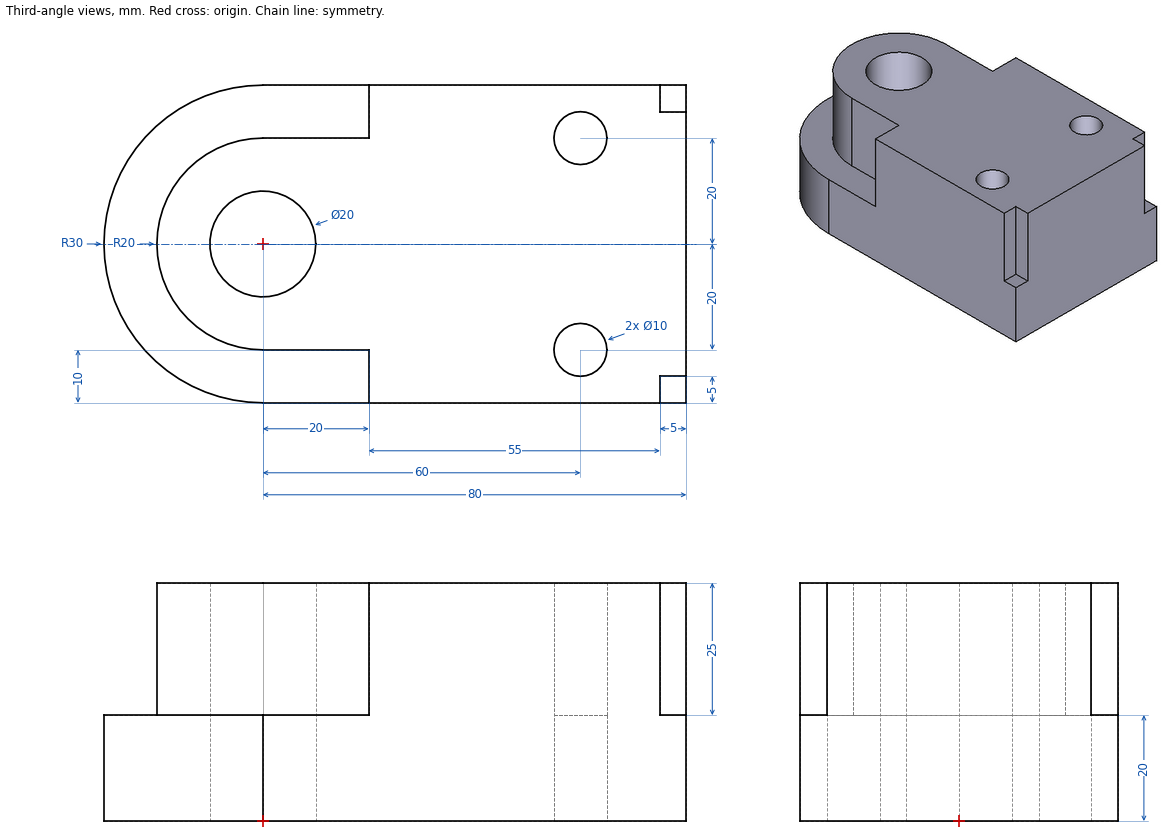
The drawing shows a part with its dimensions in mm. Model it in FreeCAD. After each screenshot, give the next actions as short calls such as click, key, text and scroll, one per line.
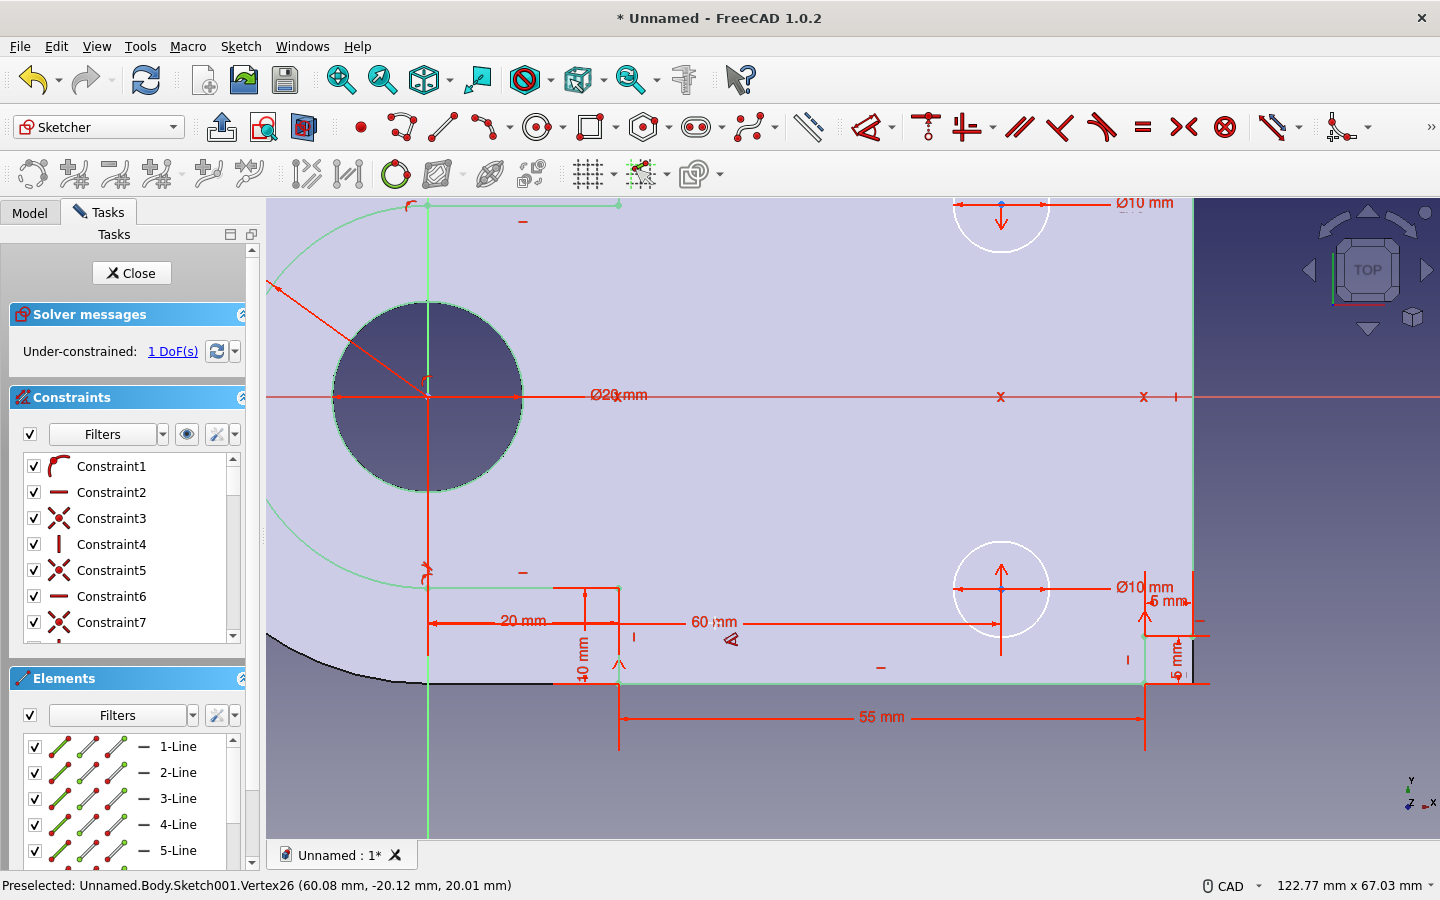
click(1001, 589)
click(1035, 493)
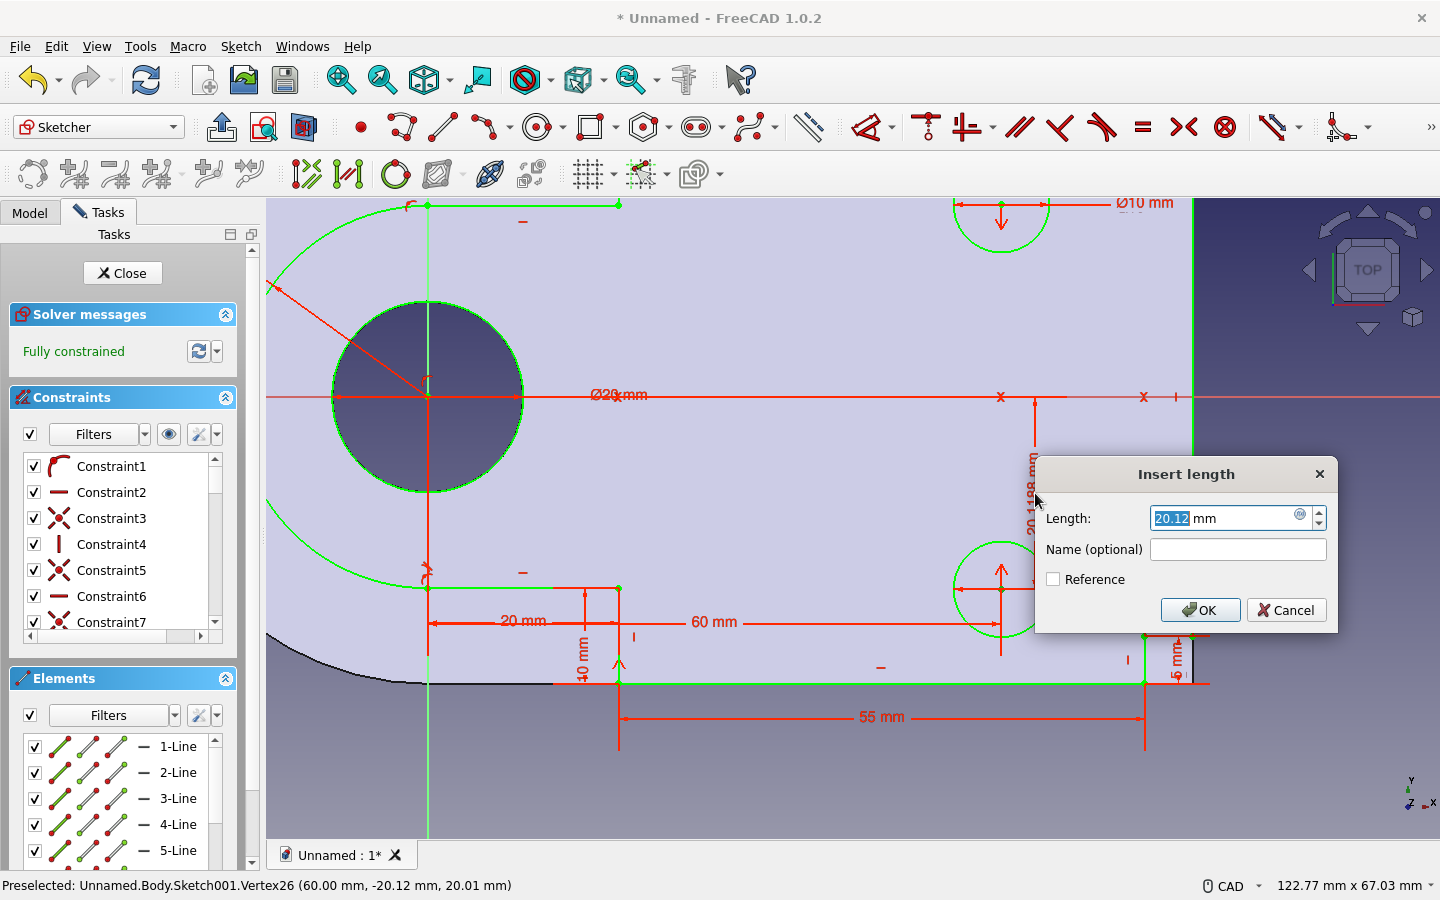
text(20)
key(Return)
key(Escape)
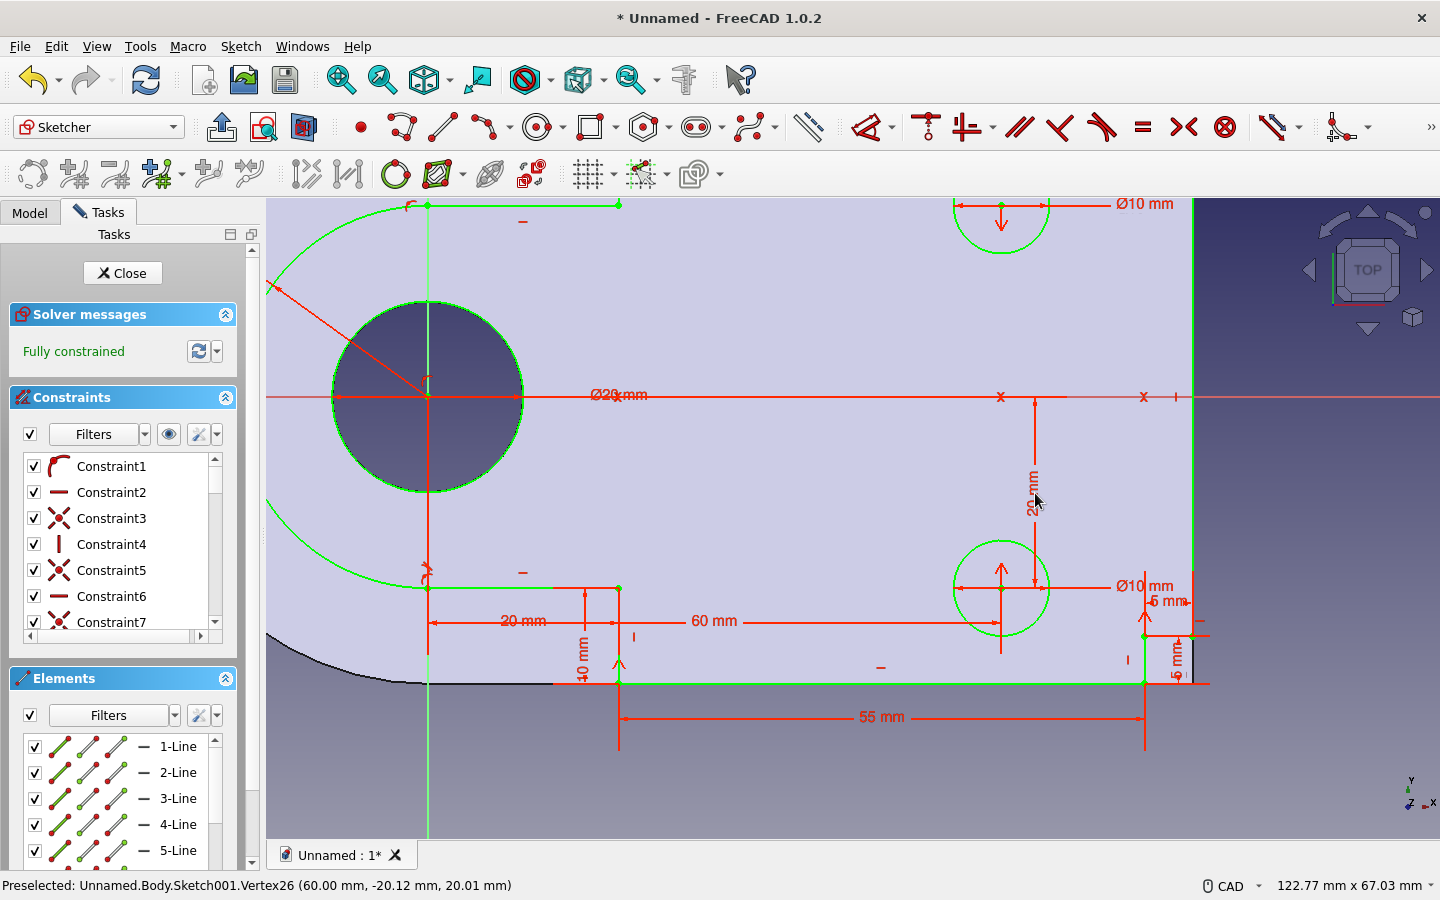
click(123, 273)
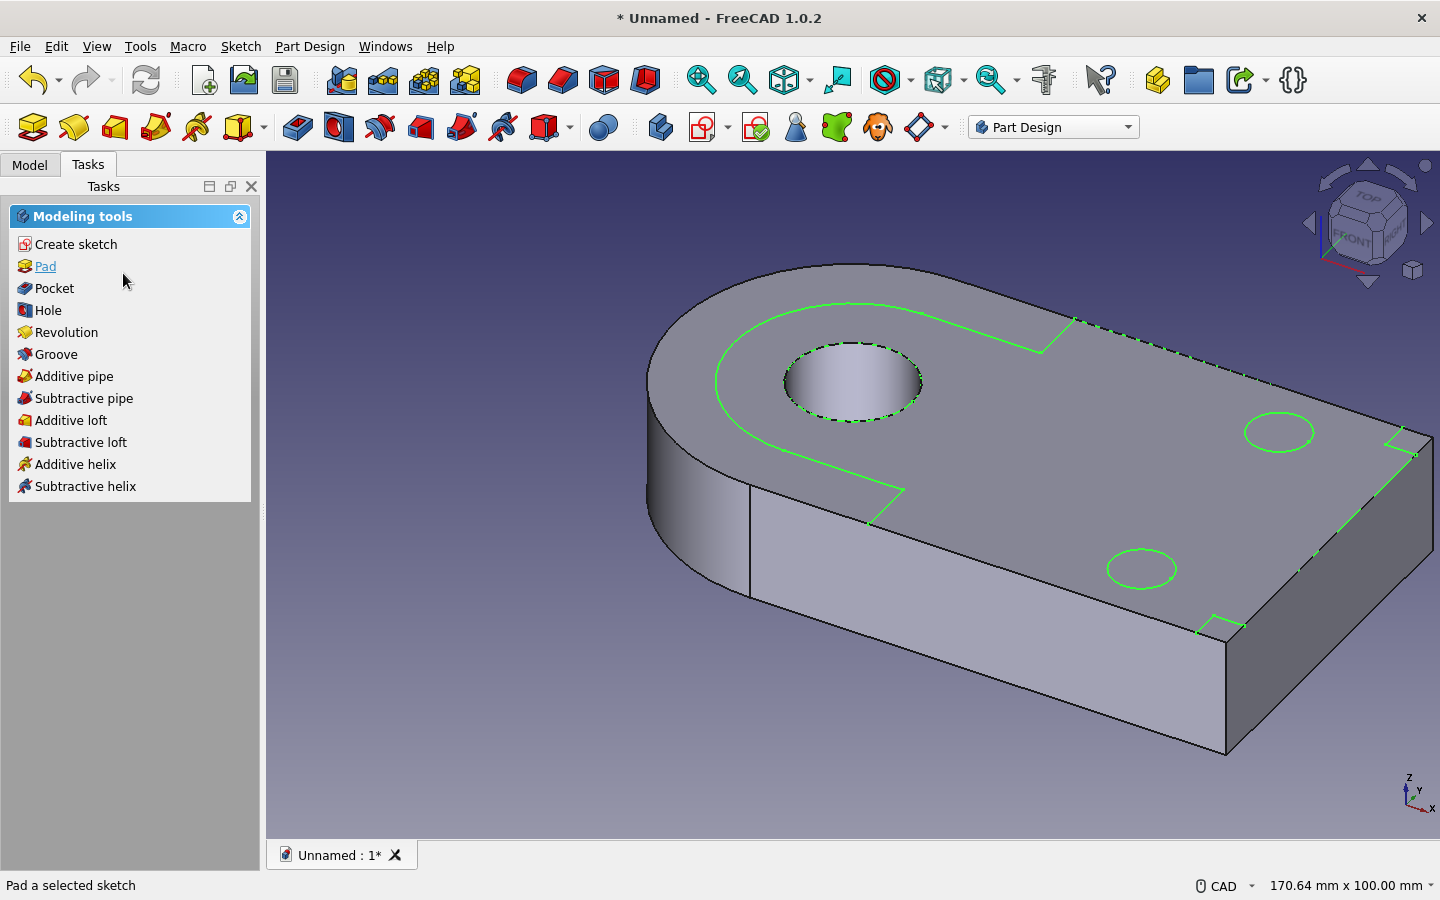
click(33, 128)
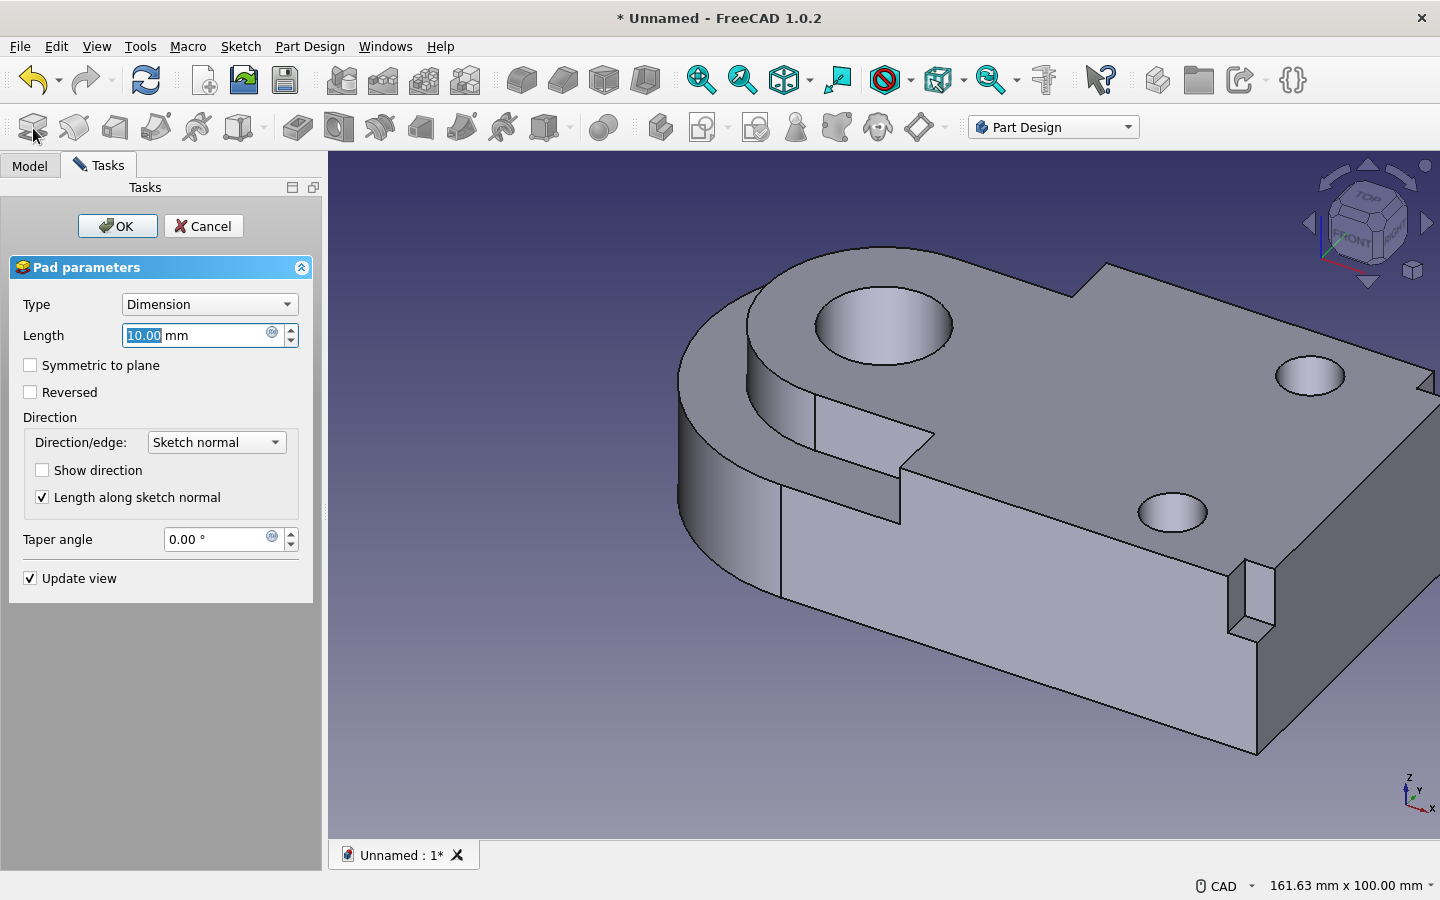
text(25)
key(Tab)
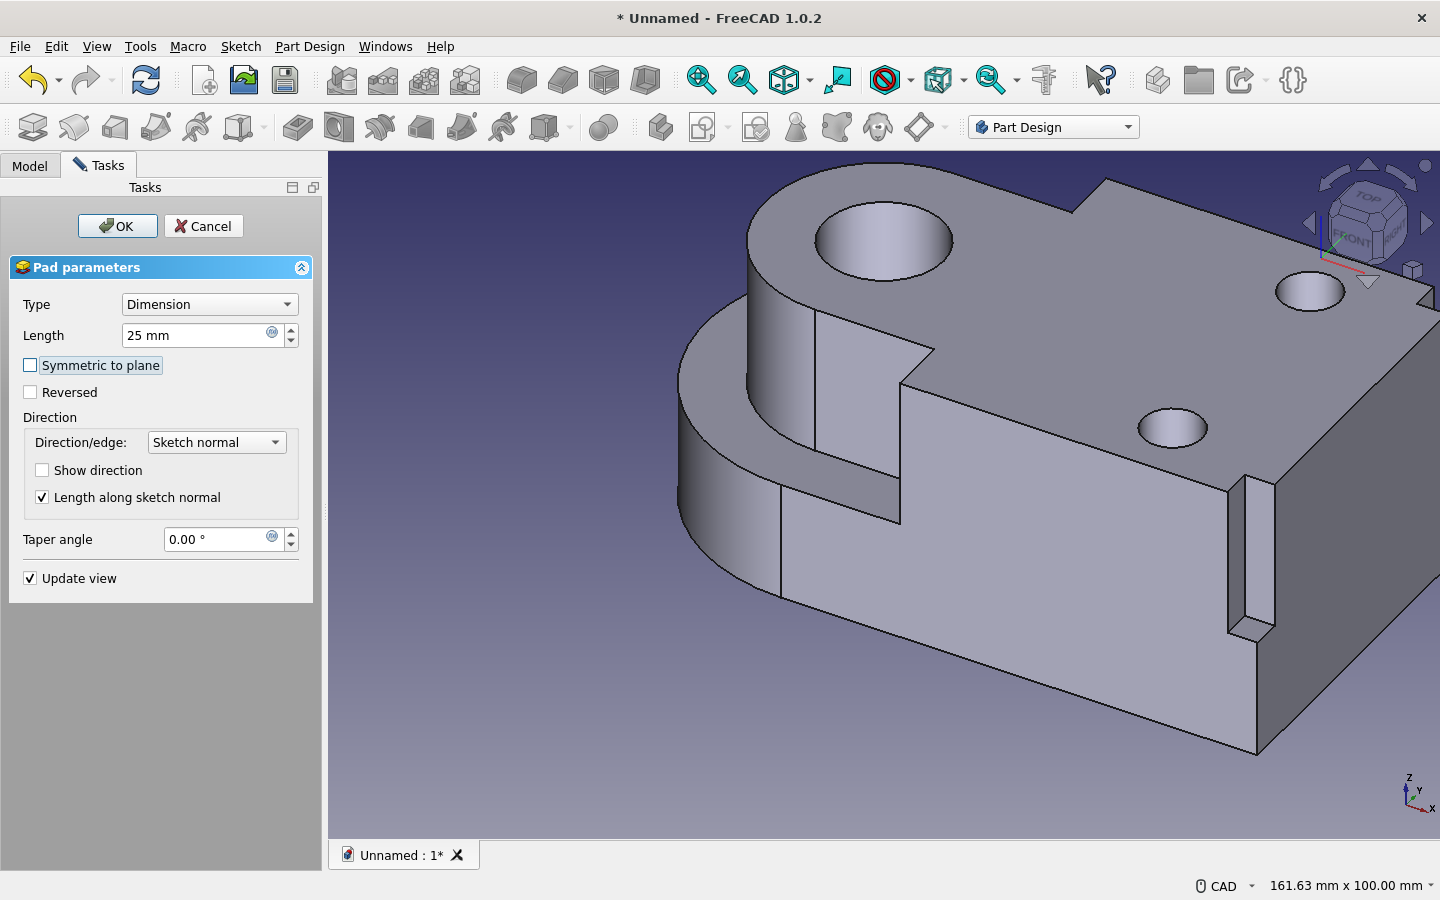
click(118, 226)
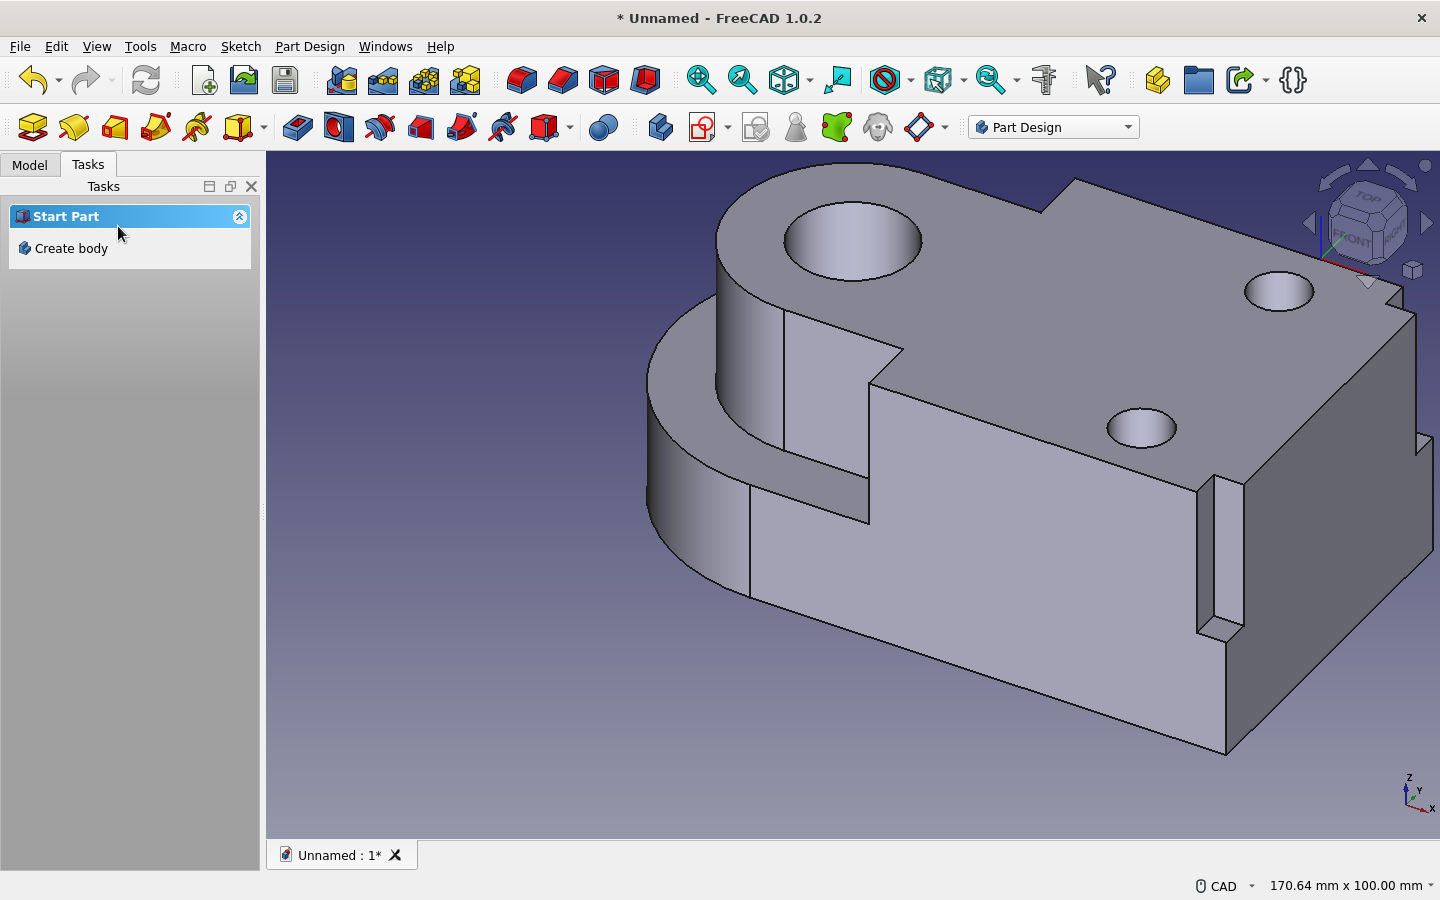
key(v)
key(f)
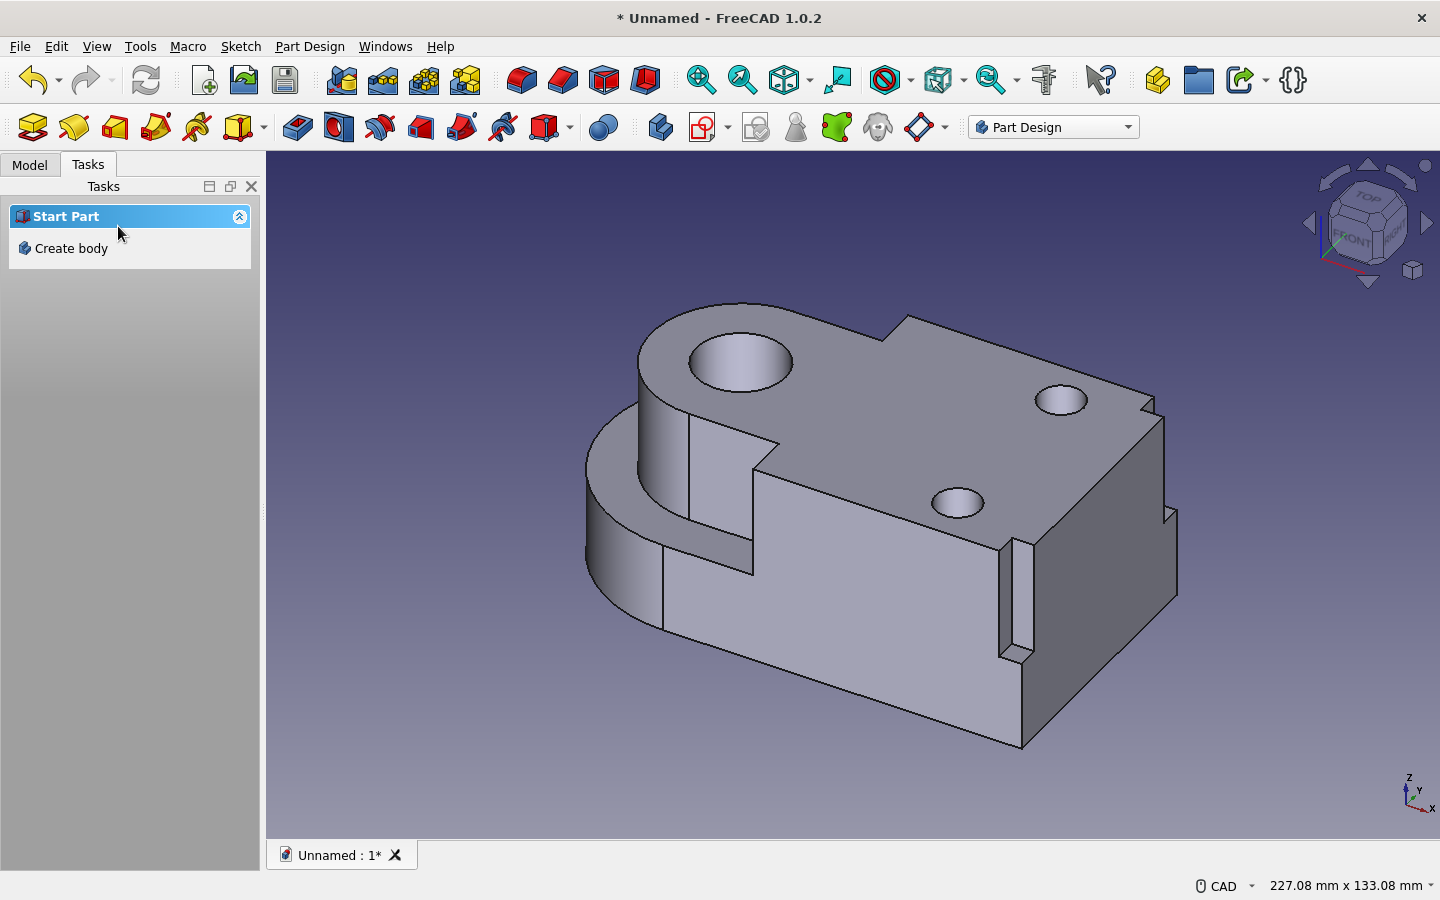
click(939, 427)